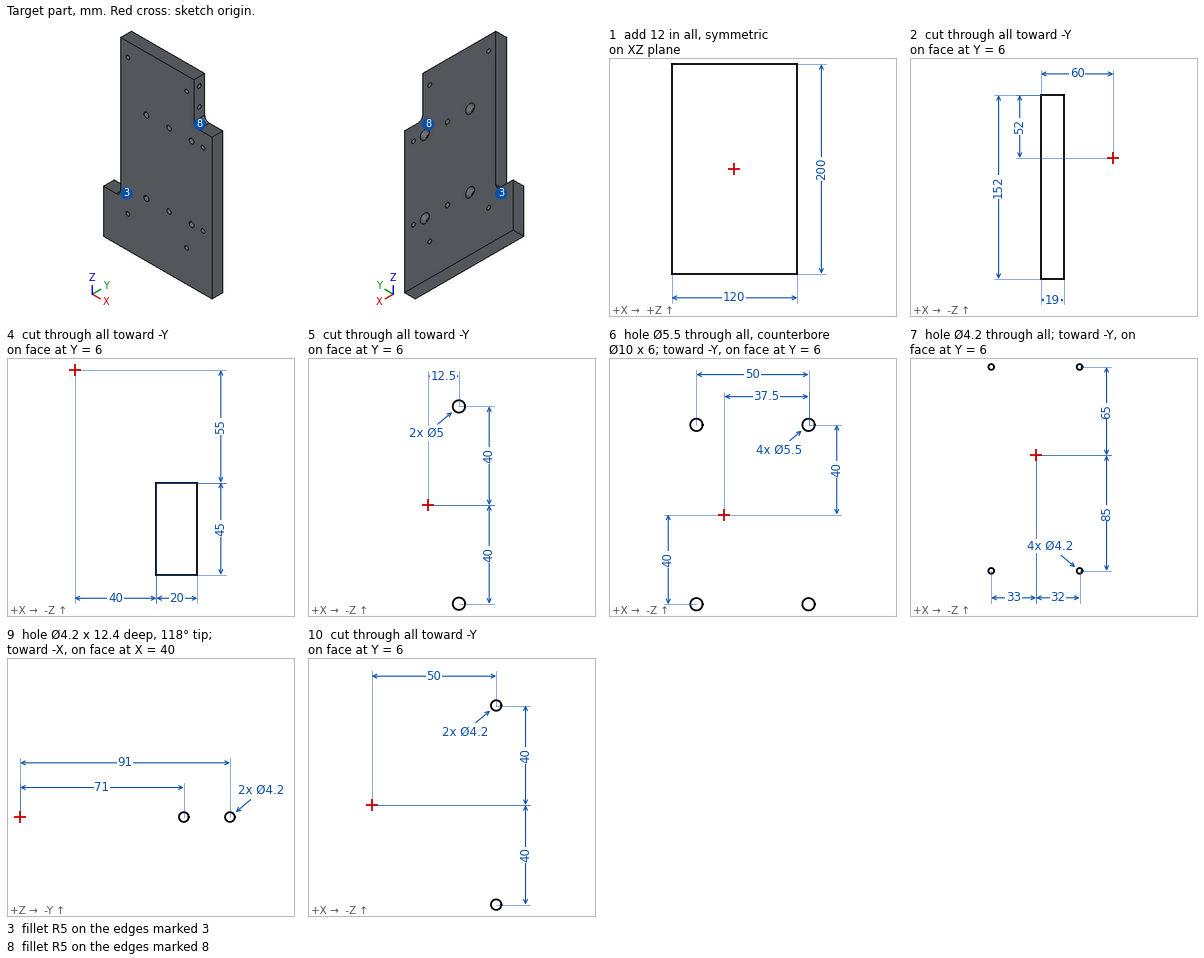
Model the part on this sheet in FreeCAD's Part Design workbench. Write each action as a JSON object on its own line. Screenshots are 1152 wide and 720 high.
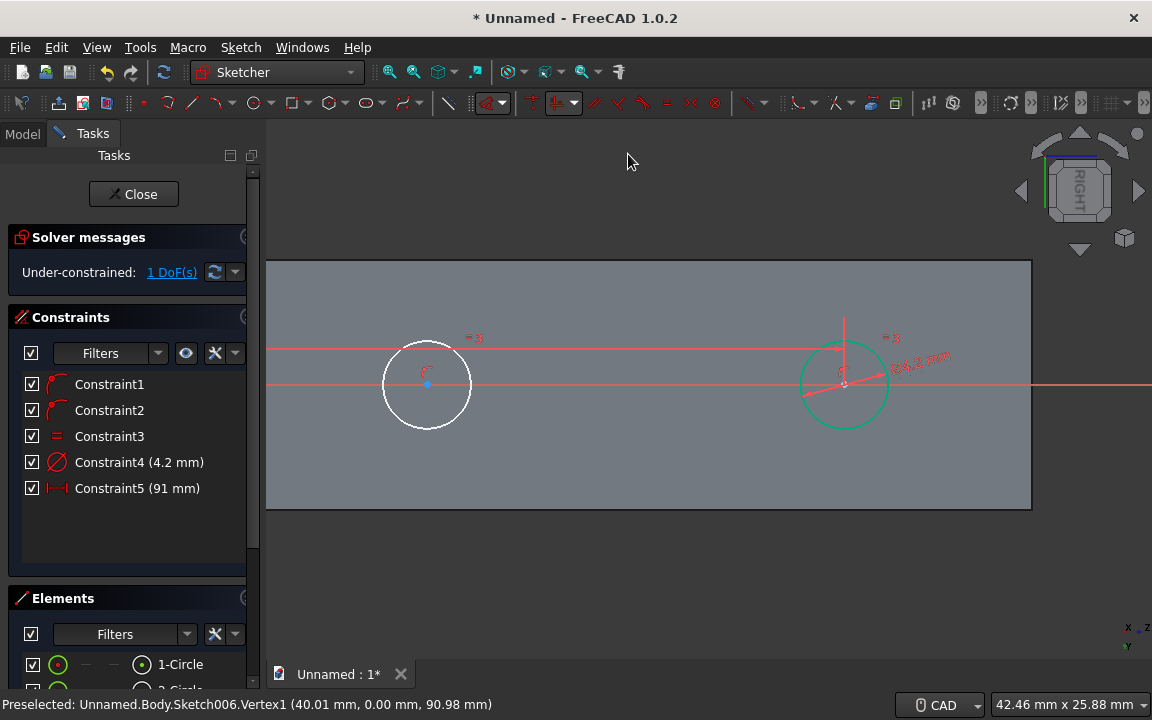
{"action": "left_click", "coordinate": [427, 385]}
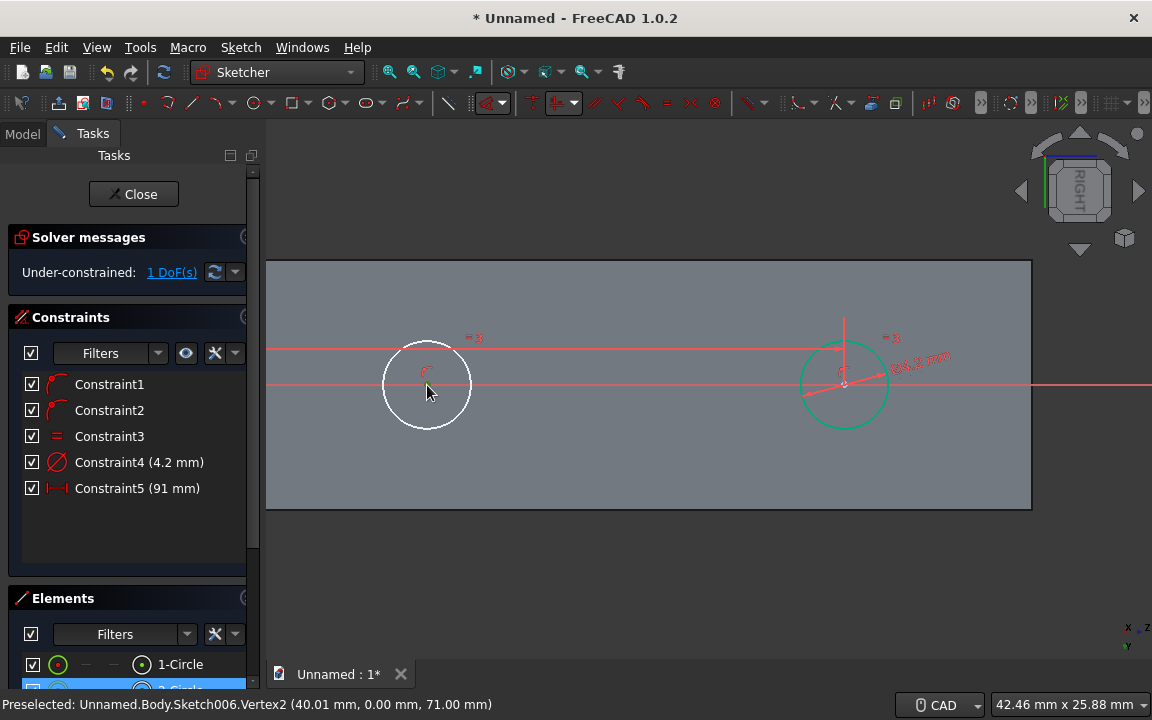
{"action": "key", "text": "l"}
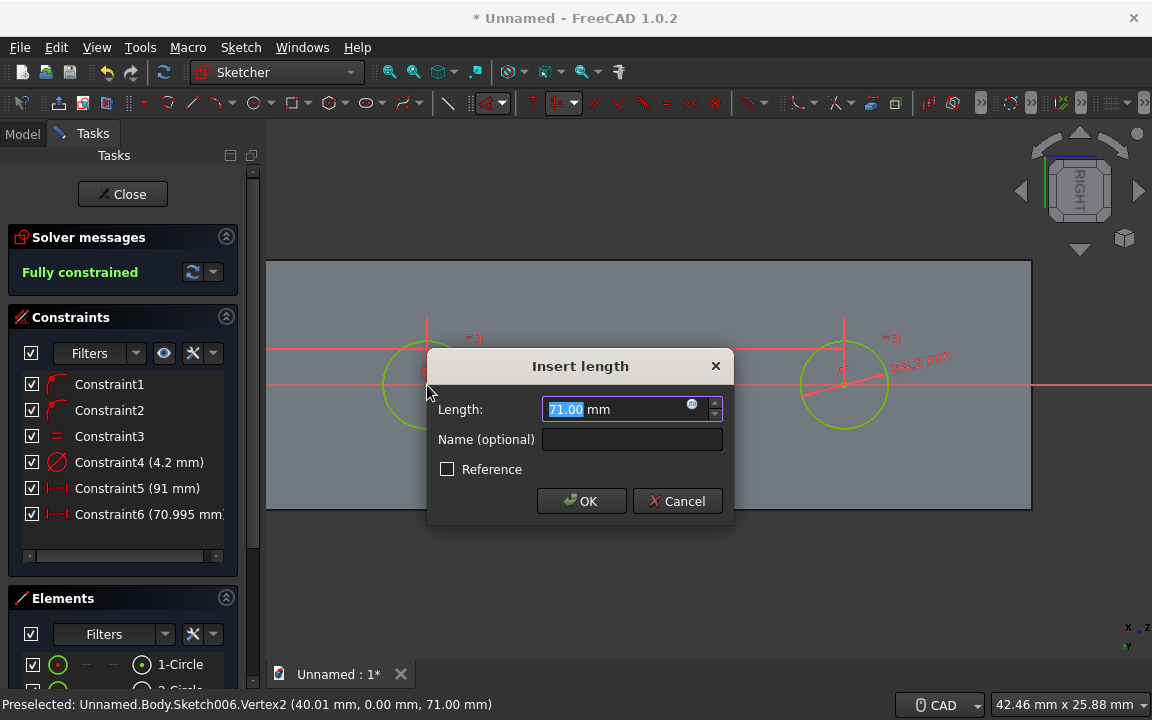
{"action": "type", "text": "71"}
{"action": "key", "text": "Return"}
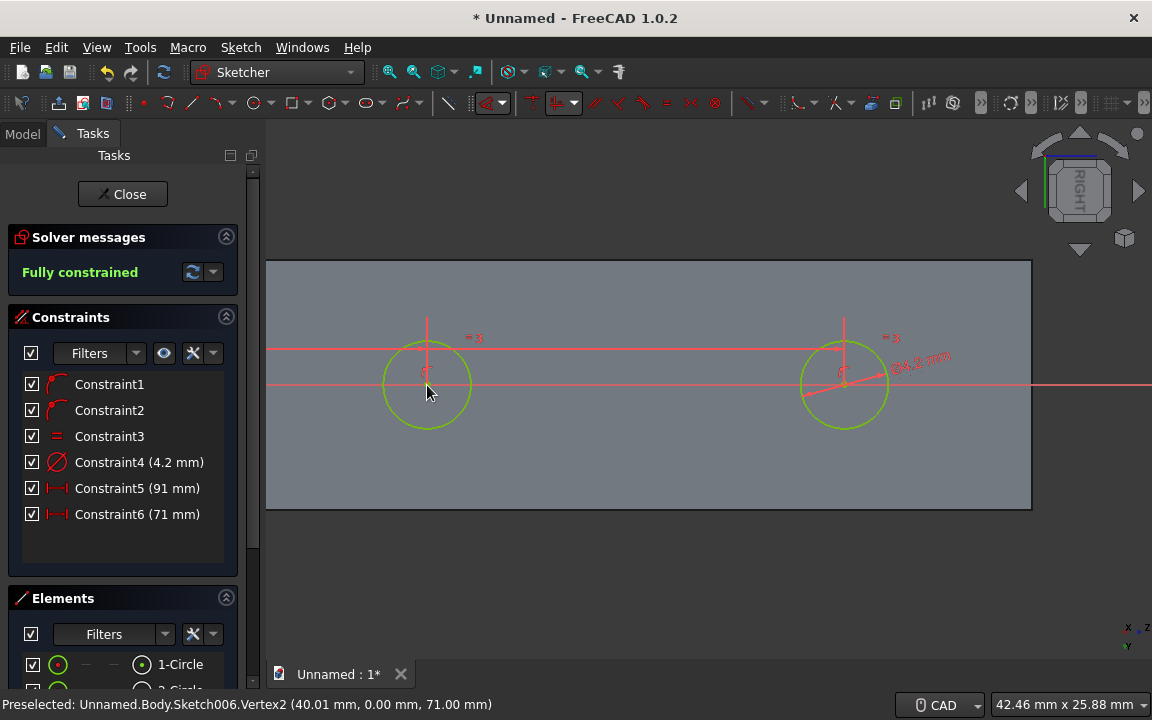
{"action": "left_click", "coordinate": [123, 194]}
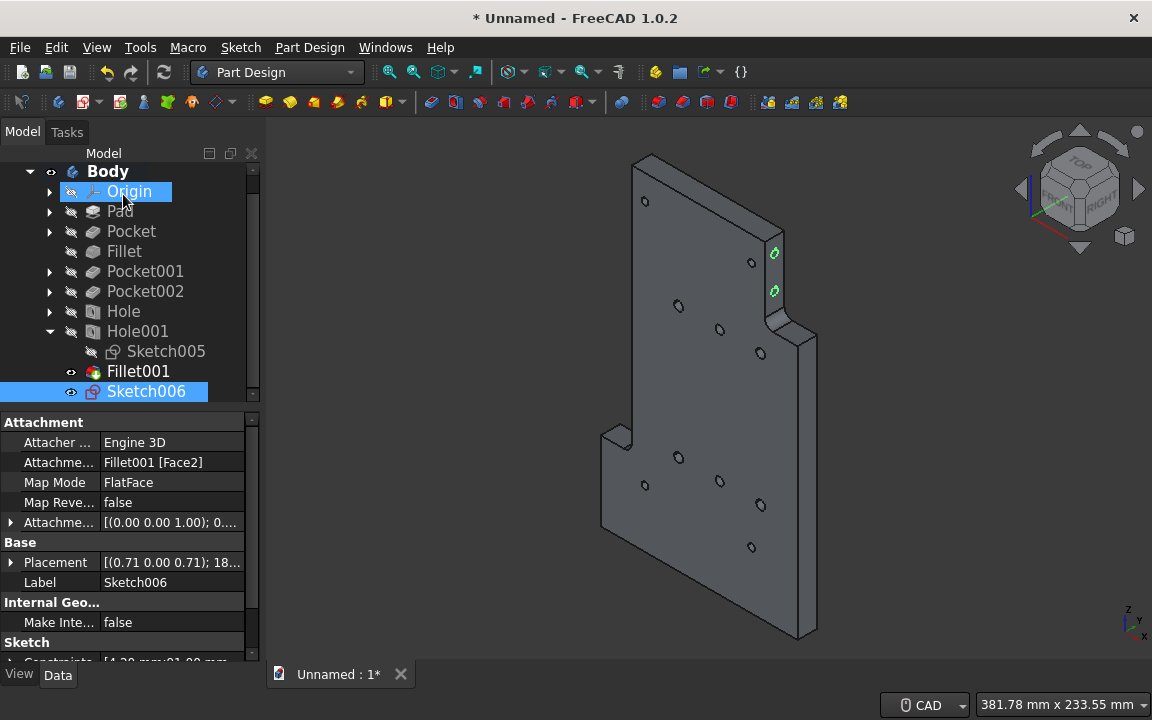
{"action": "left_click", "coordinate": [456, 102]}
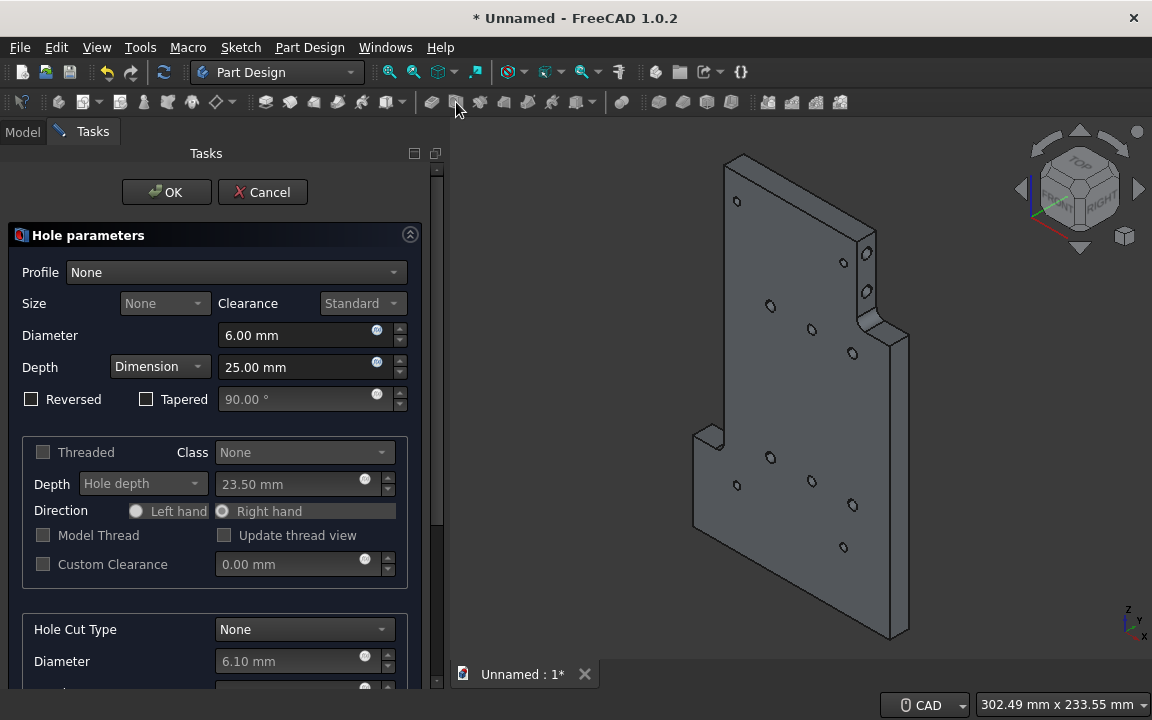
{"action": "triple_click", "coordinate": [305, 335]}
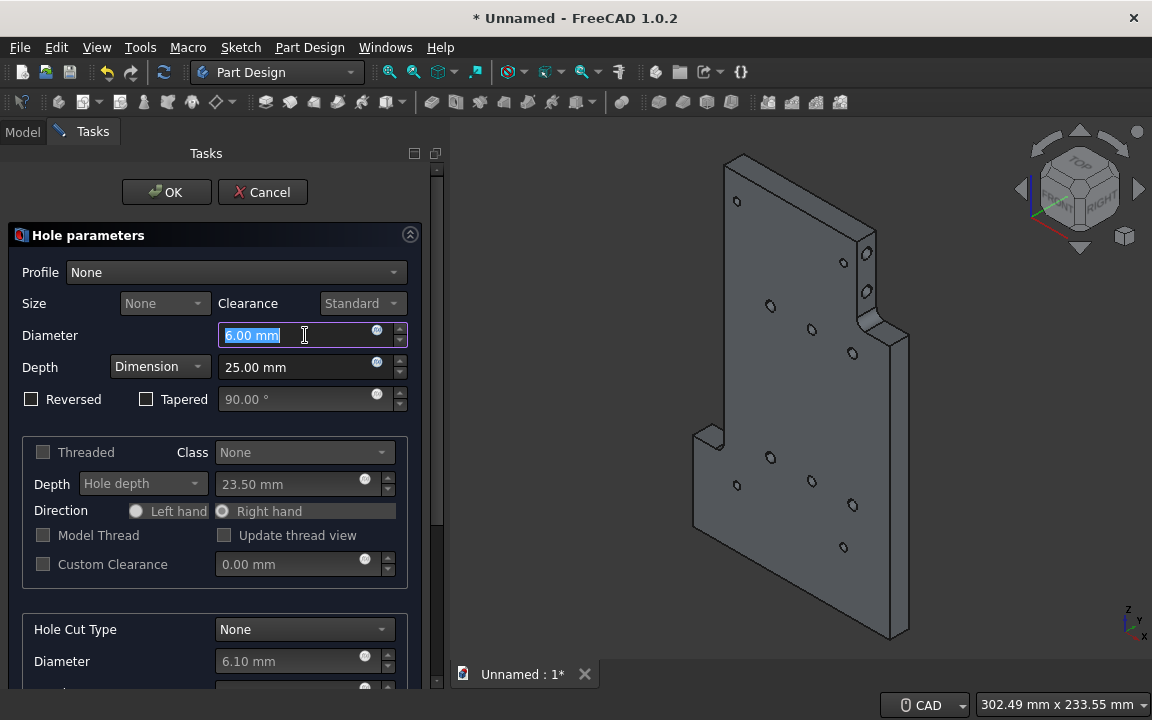
{"action": "type", "text": "4.2"}
{"action": "key", "text": "Tab"}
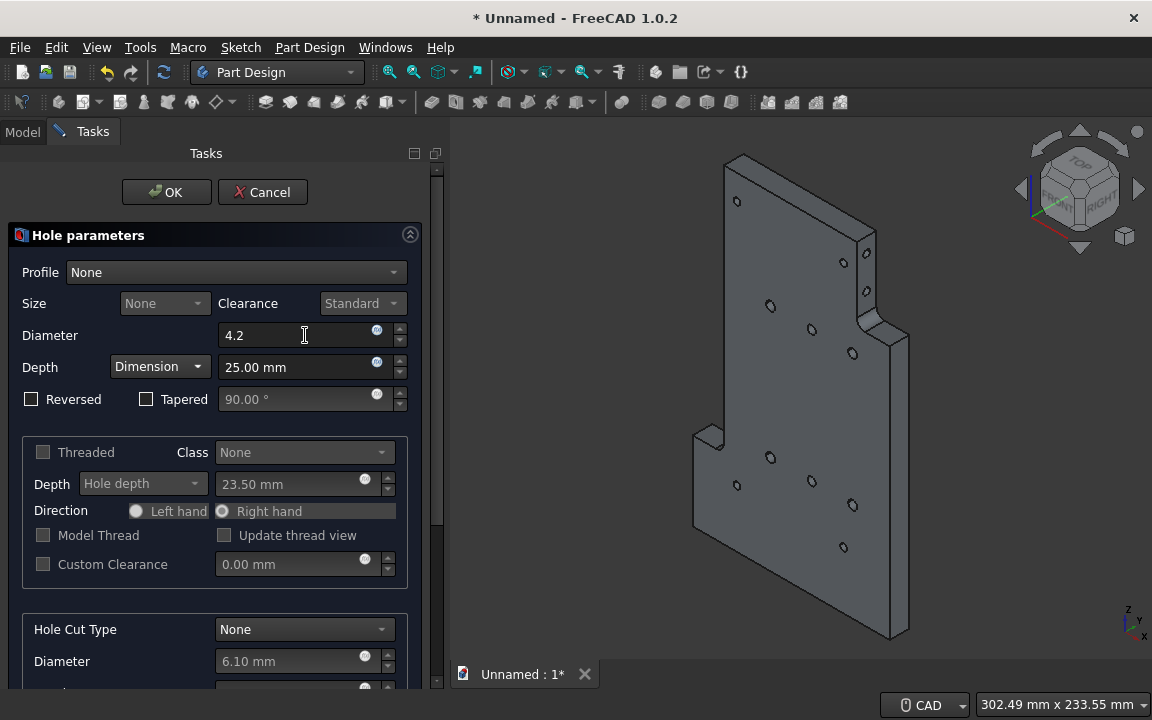
{"action": "triple_click", "coordinate": [305, 367]}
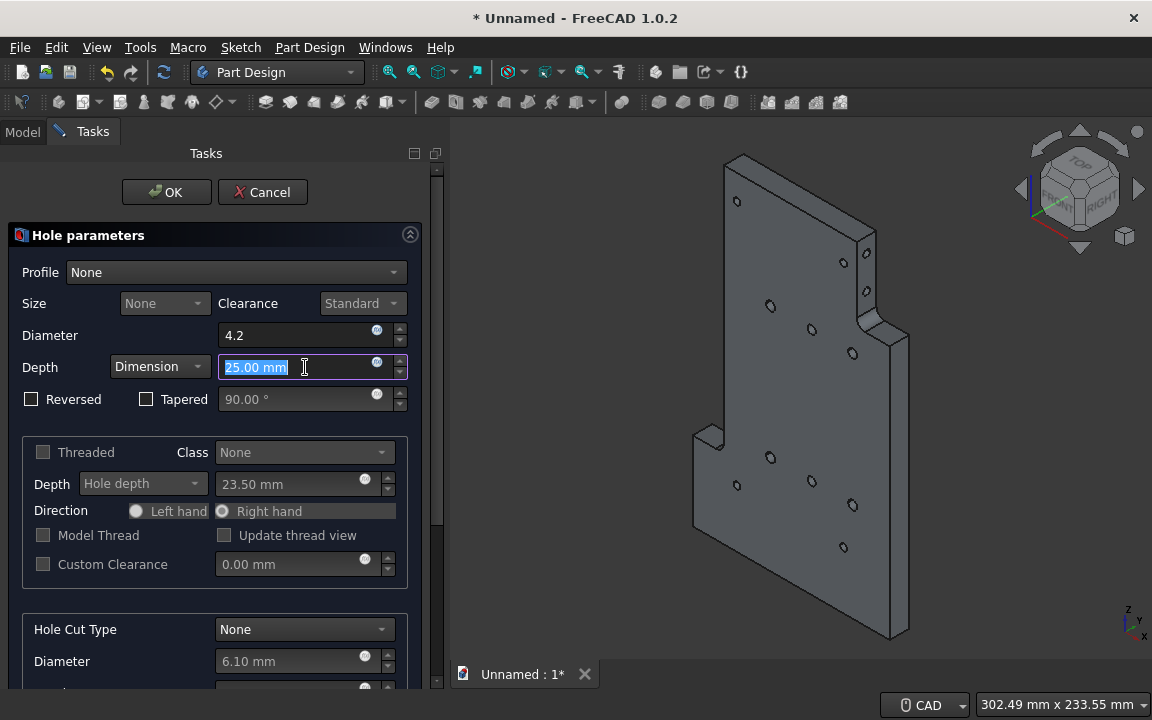
{"action": "type", "text": "12.4"}
{"action": "key", "text": "Tab"}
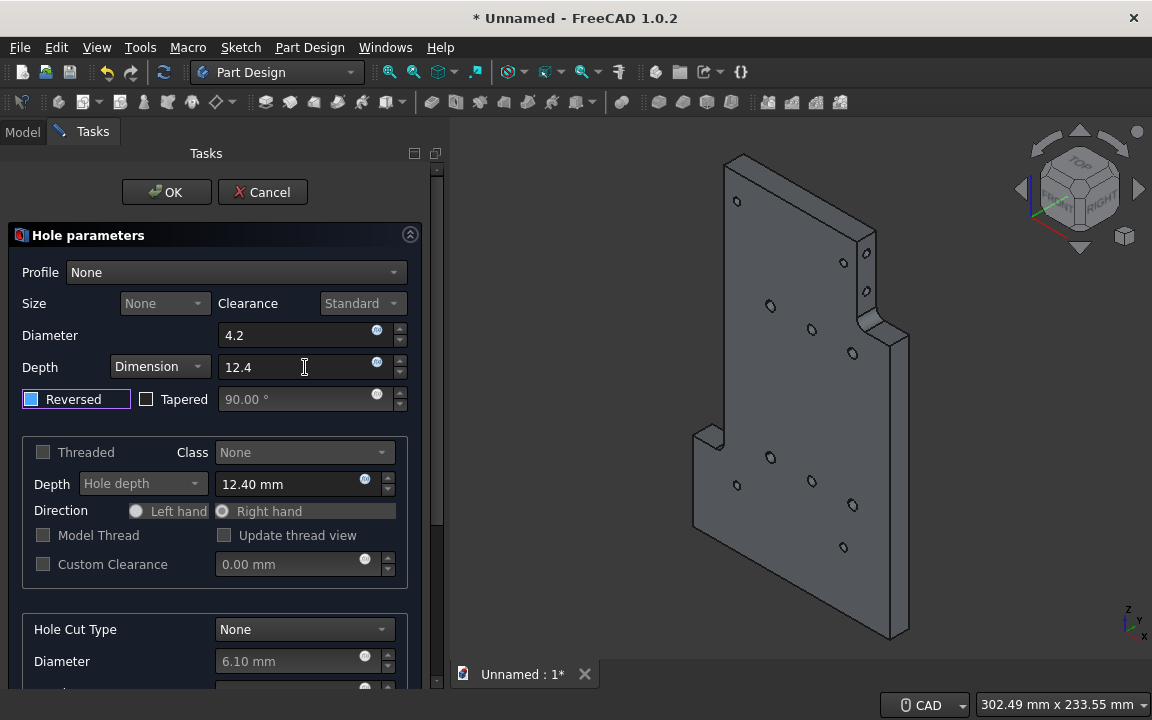
{"action": "left_click", "coordinate": [167, 192]}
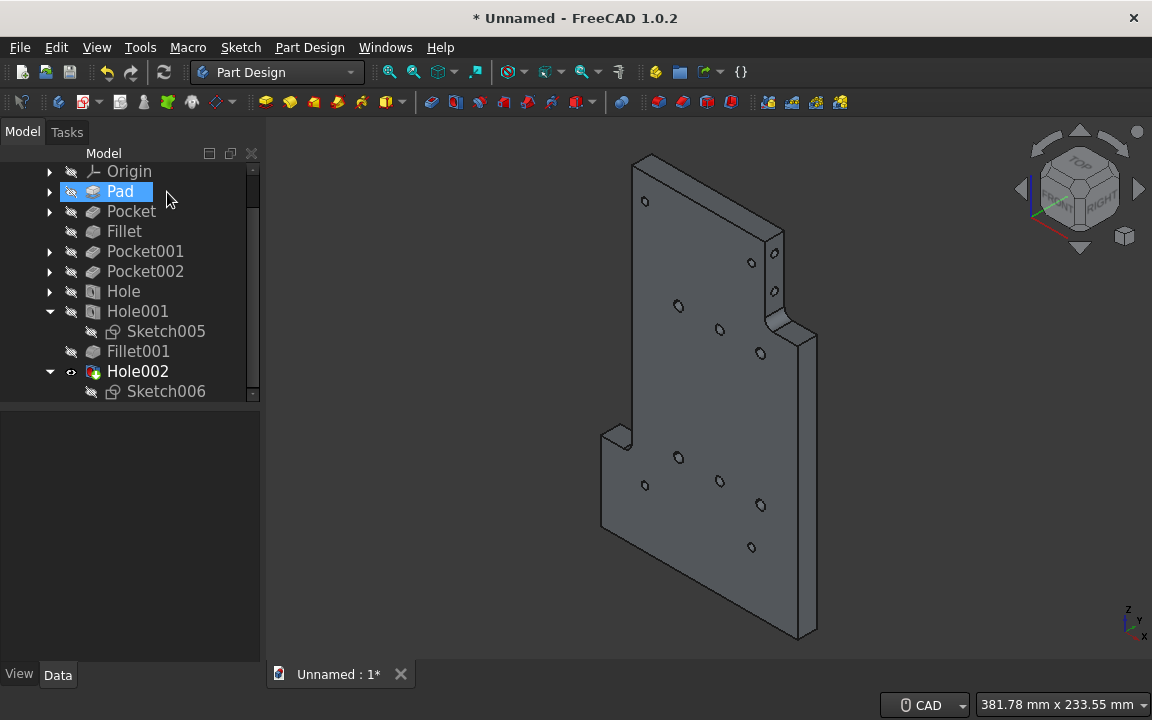
{"action": "key", "text": "4"}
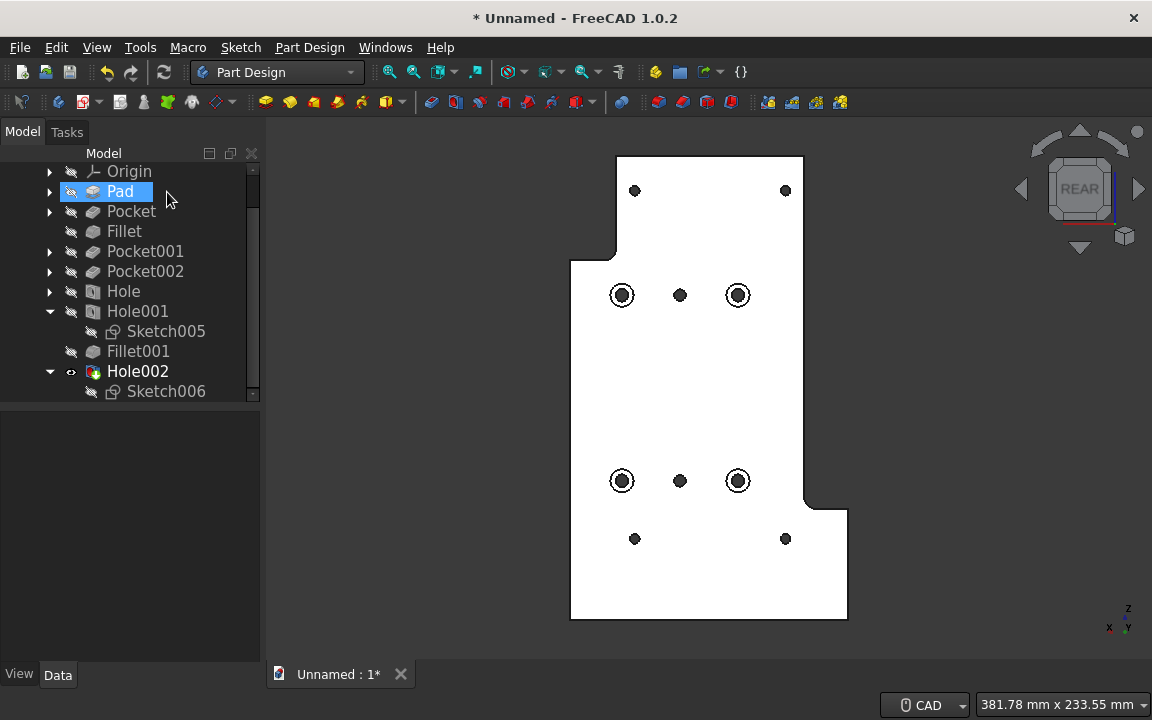
{"action": "left_click", "coordinate": [669, 387]}